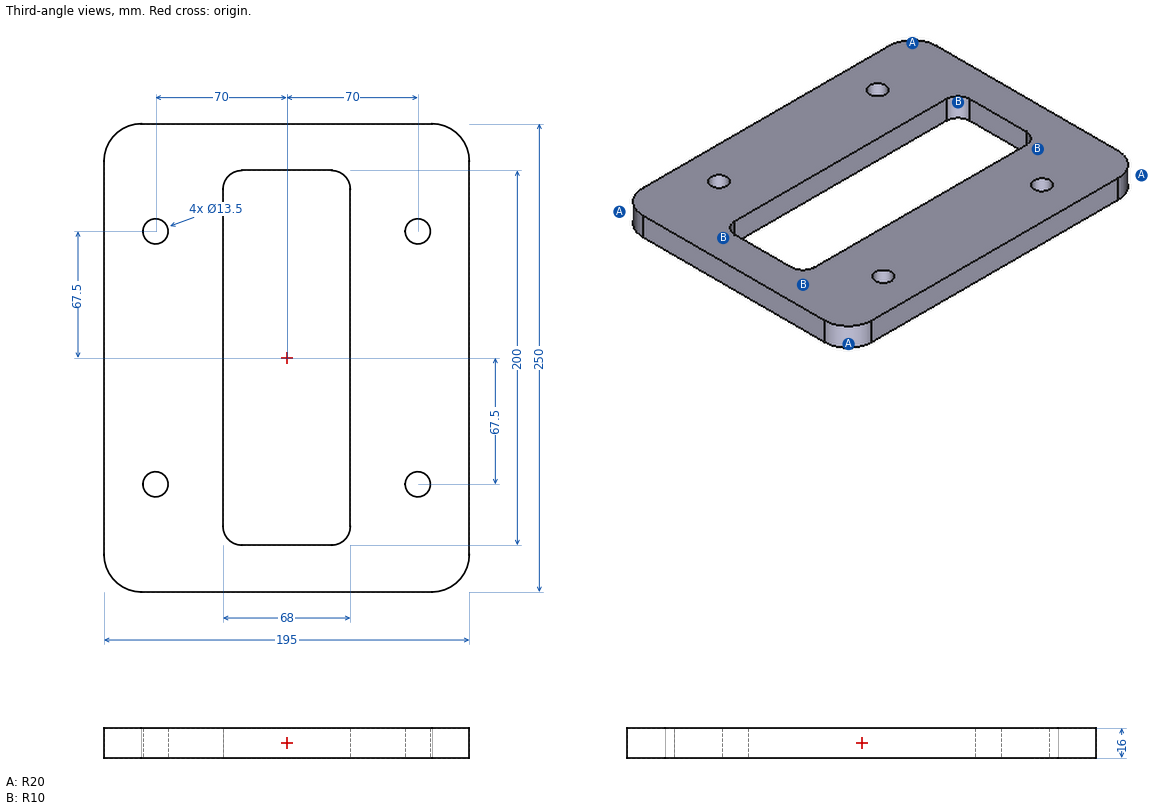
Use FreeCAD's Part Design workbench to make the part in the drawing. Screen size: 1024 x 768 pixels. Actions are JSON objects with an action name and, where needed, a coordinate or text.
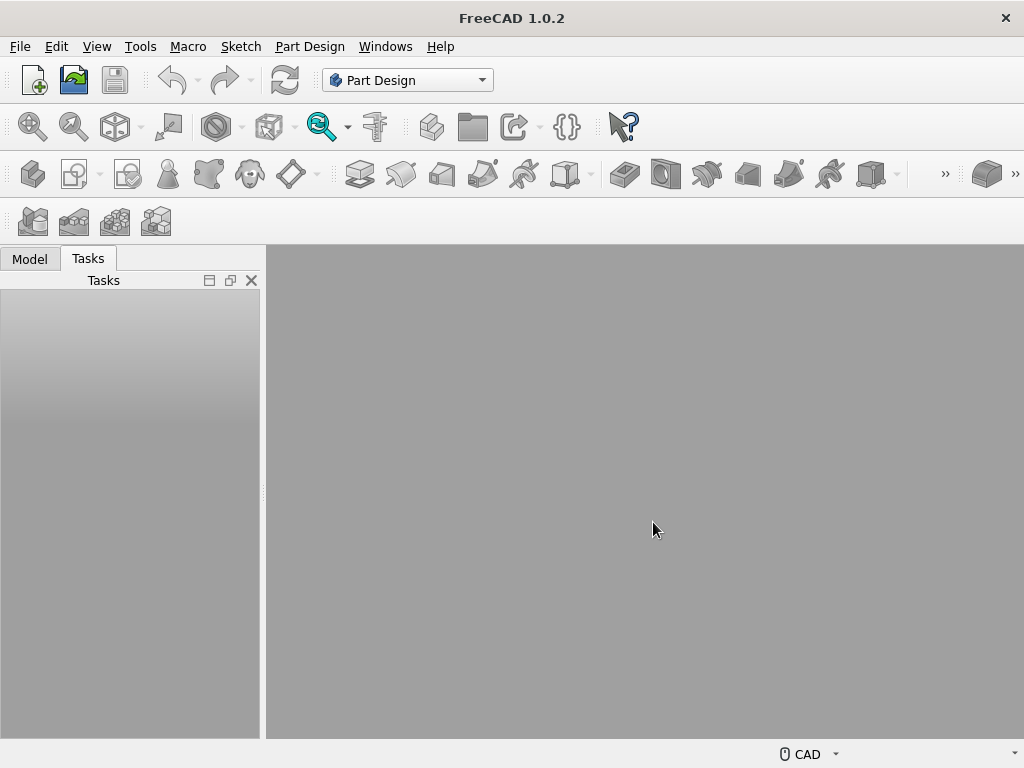
{"action": "left_click", "coordinate": [33, 80]}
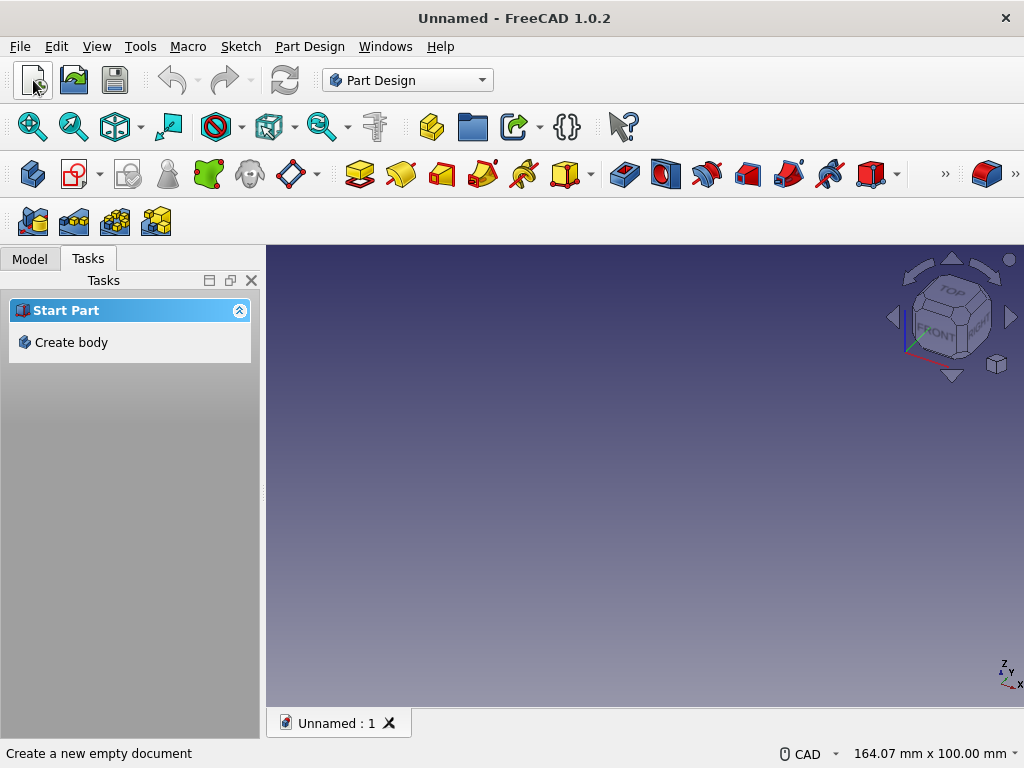
{"action": "left_click", "coordinate": [74, 174]}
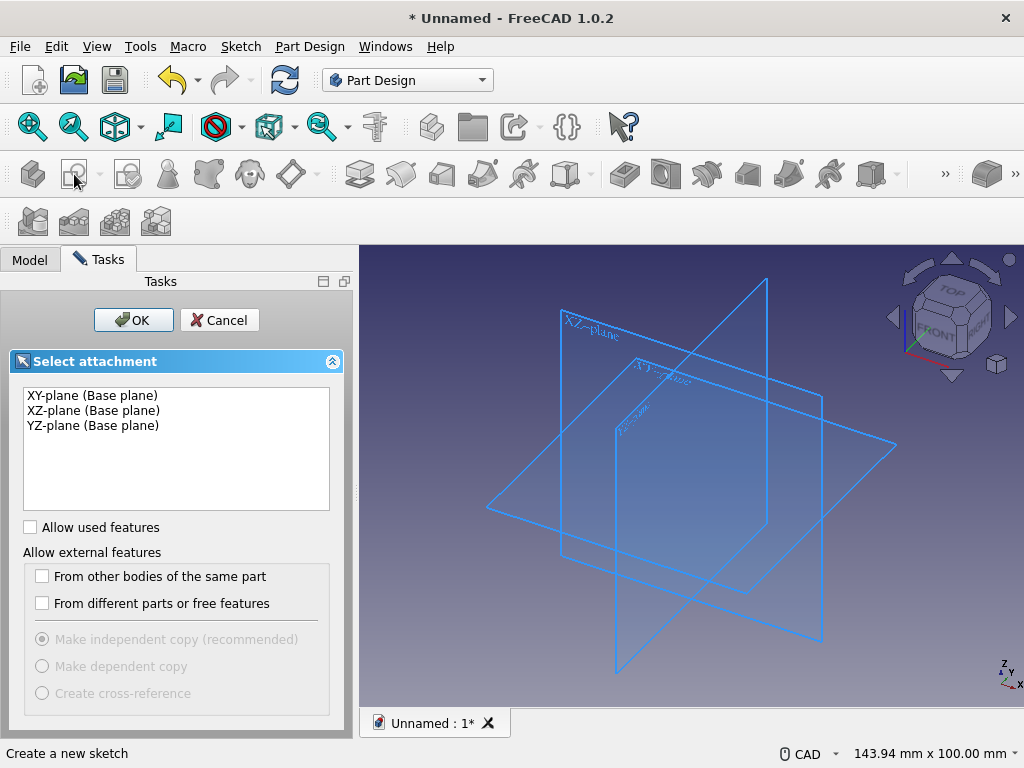
{"action": "left_click", "coordinate": [84, 396]}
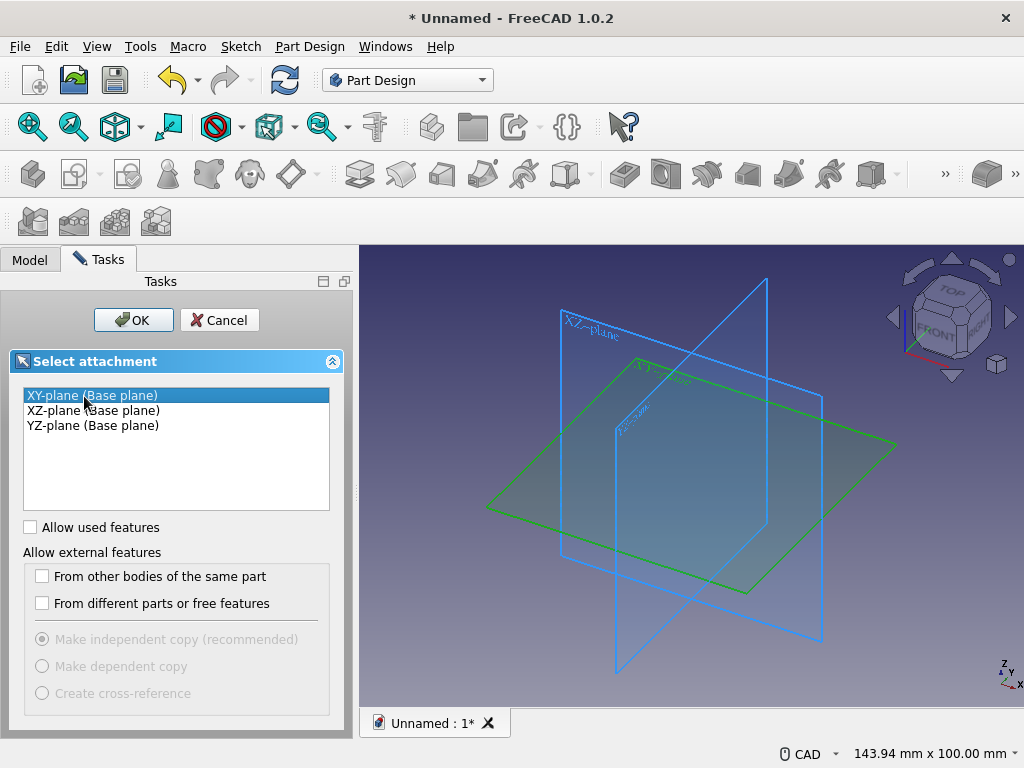
{"action": "left_click", "coordinate": [134, 320]}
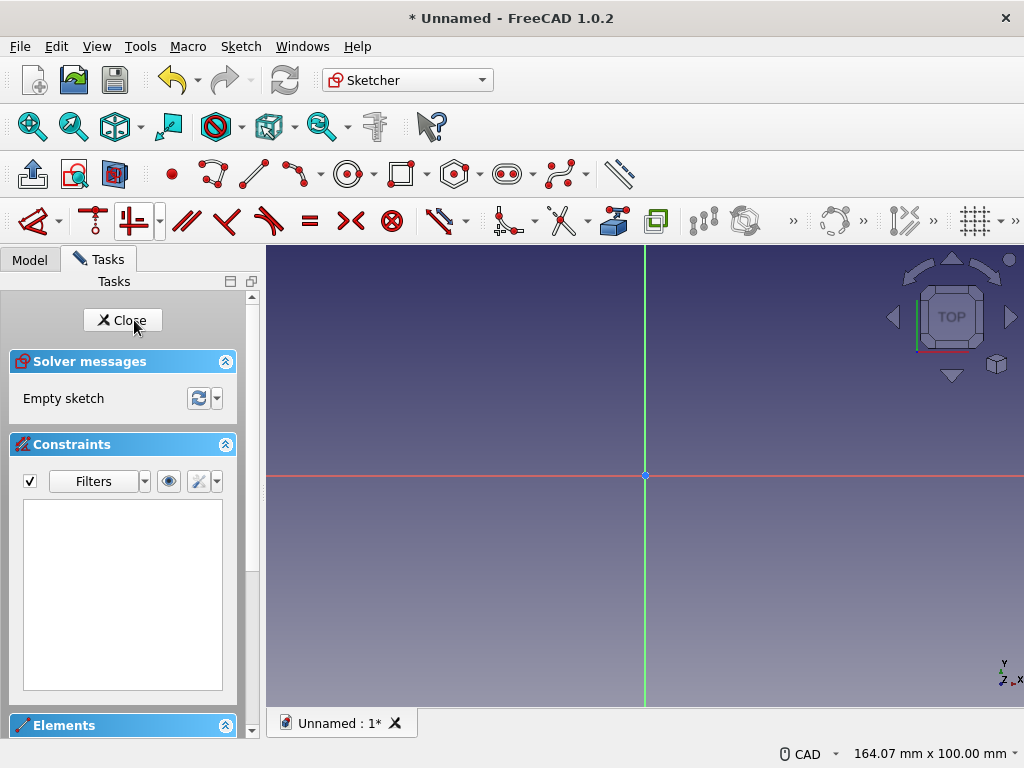
{"action": "scroll", "coordinate": [554, 476], "scroll_direction": "down", "scroll_amount": 7}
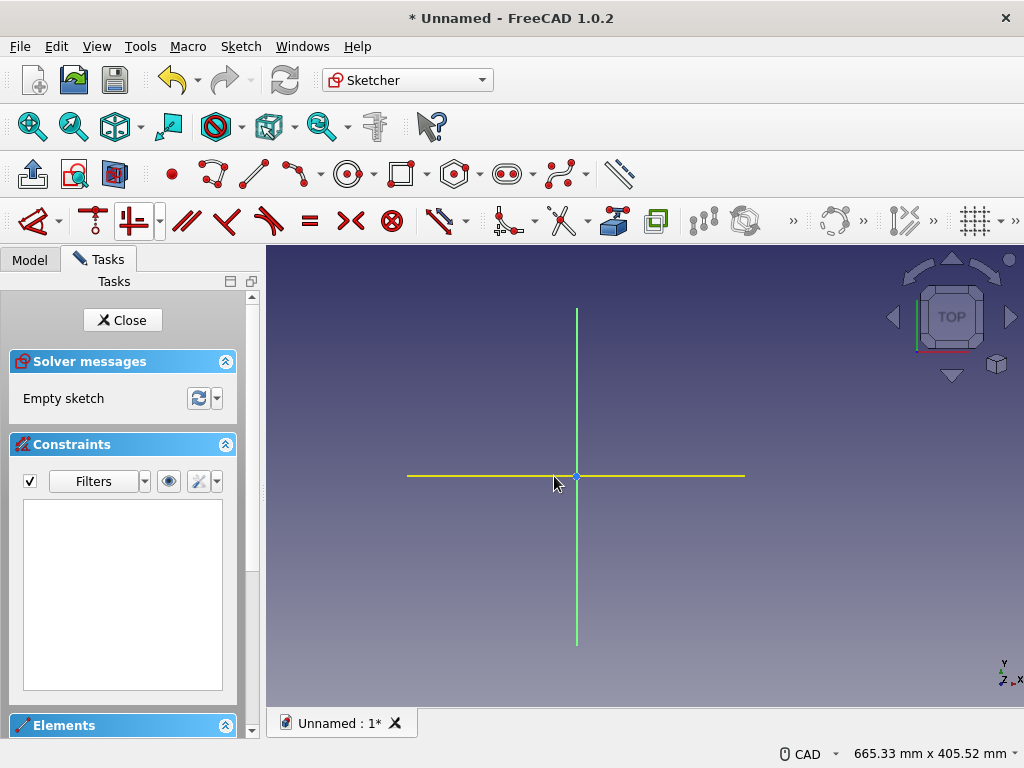
{"action": "left_click", "coordinate": [426, 174]}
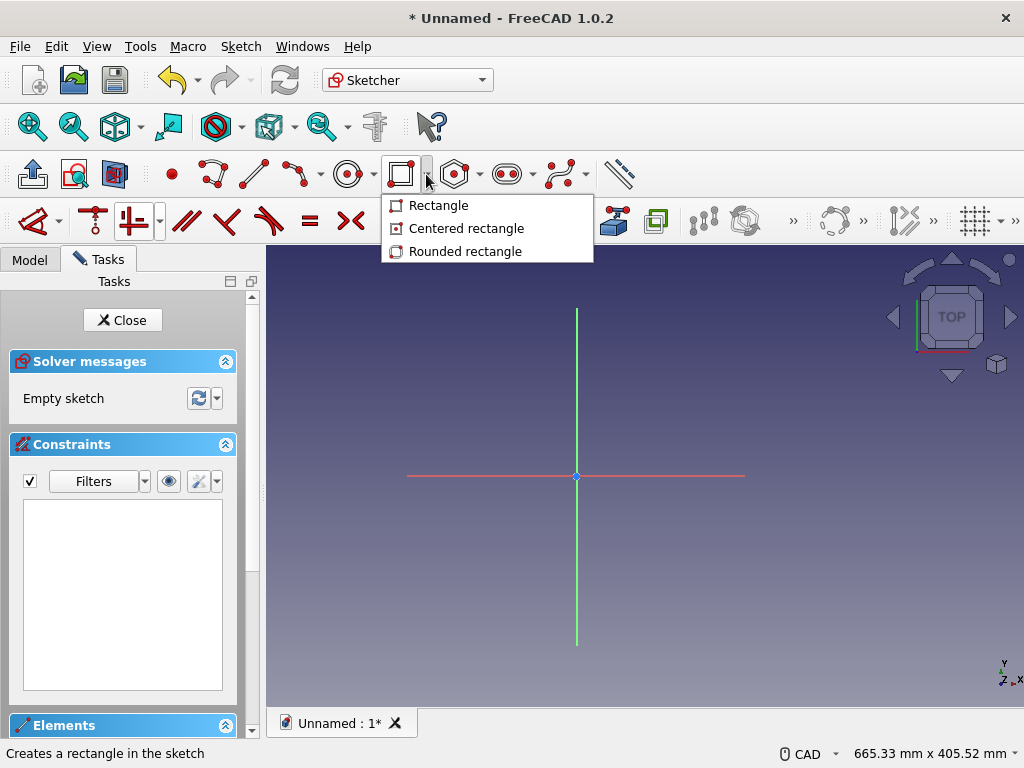
{"action": "left_click", "coordinate": [488, 228]}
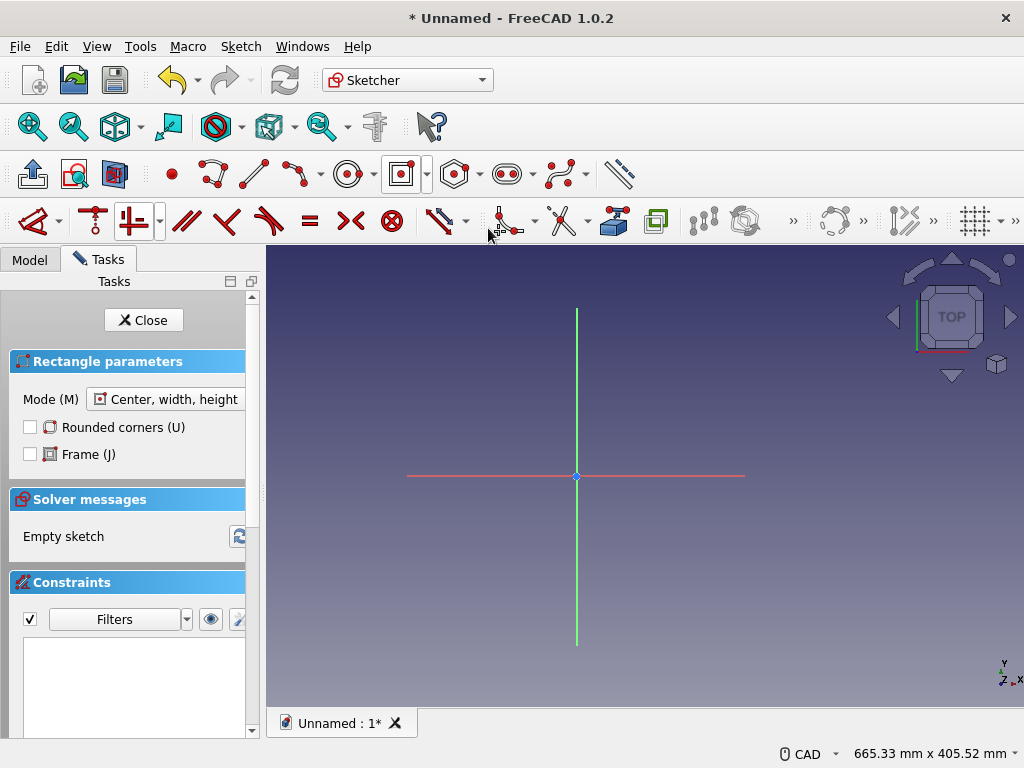
{"action": "left_click", "coordinate": [577, 476]}
{"action": "left_click", "coordinate": [688, 334]}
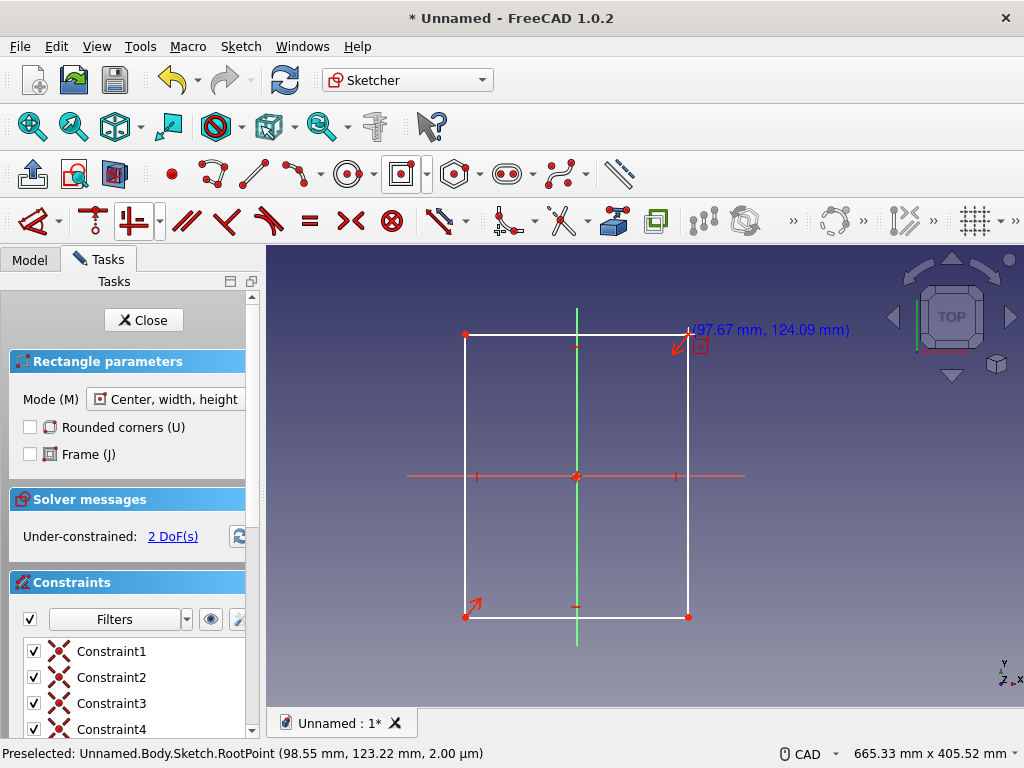
{"action": "left_click", "coordinate": [577, 476]}
{"action": "left_click", "coordinate": [615, 362]}
{"action": "key", "text": "Escape"}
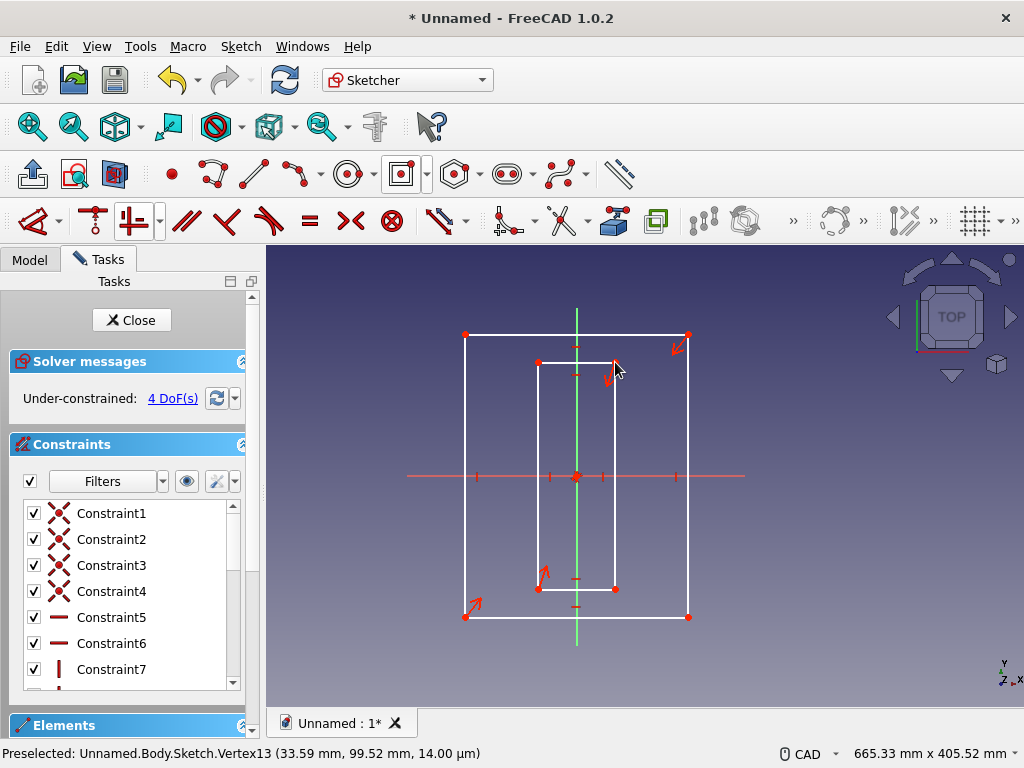
{"action": "left_click", "coordinate": [32, 222]}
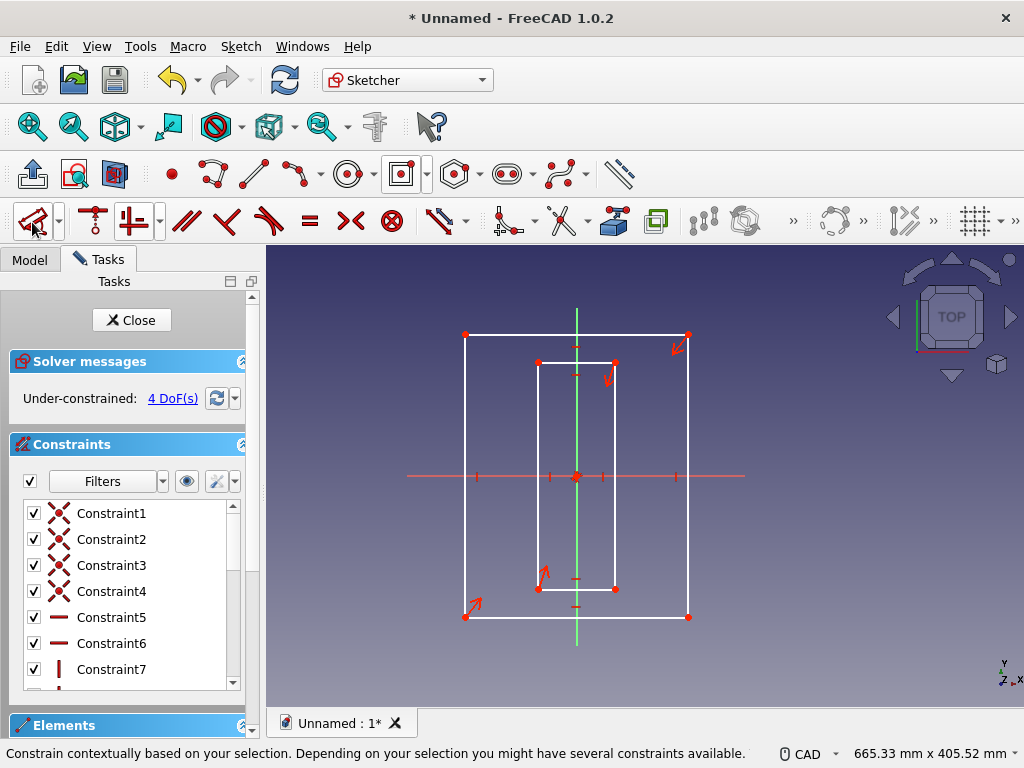
{"action": "left_click", "coordinate": [561, 590]}
{"action": "left_click", "coordinate": [559, 556]}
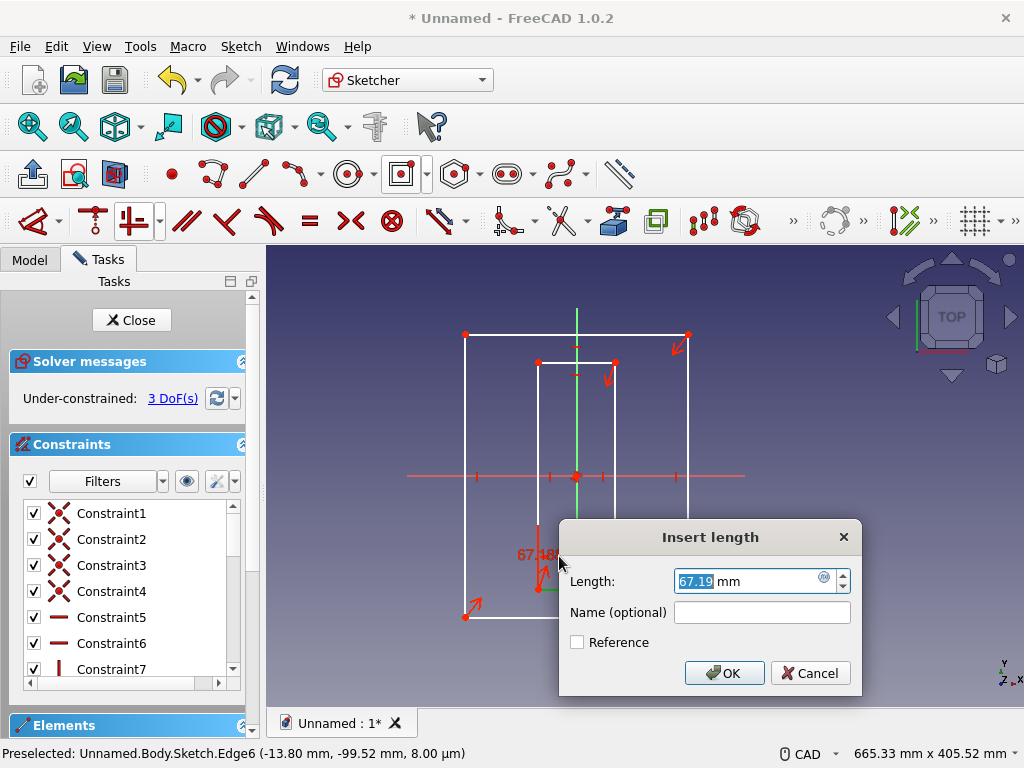
{"action": "type", "text": "68"}
{"action": "key", "text": "Return"}